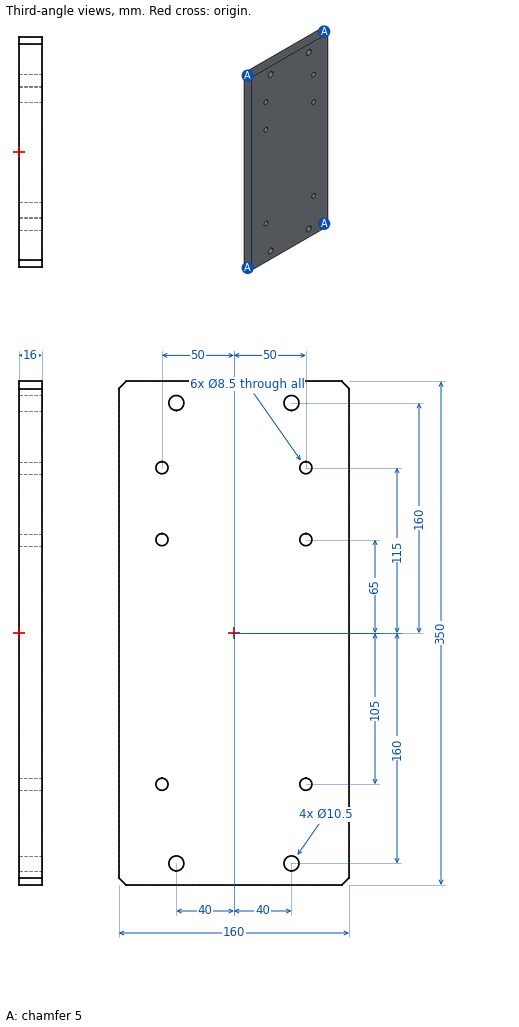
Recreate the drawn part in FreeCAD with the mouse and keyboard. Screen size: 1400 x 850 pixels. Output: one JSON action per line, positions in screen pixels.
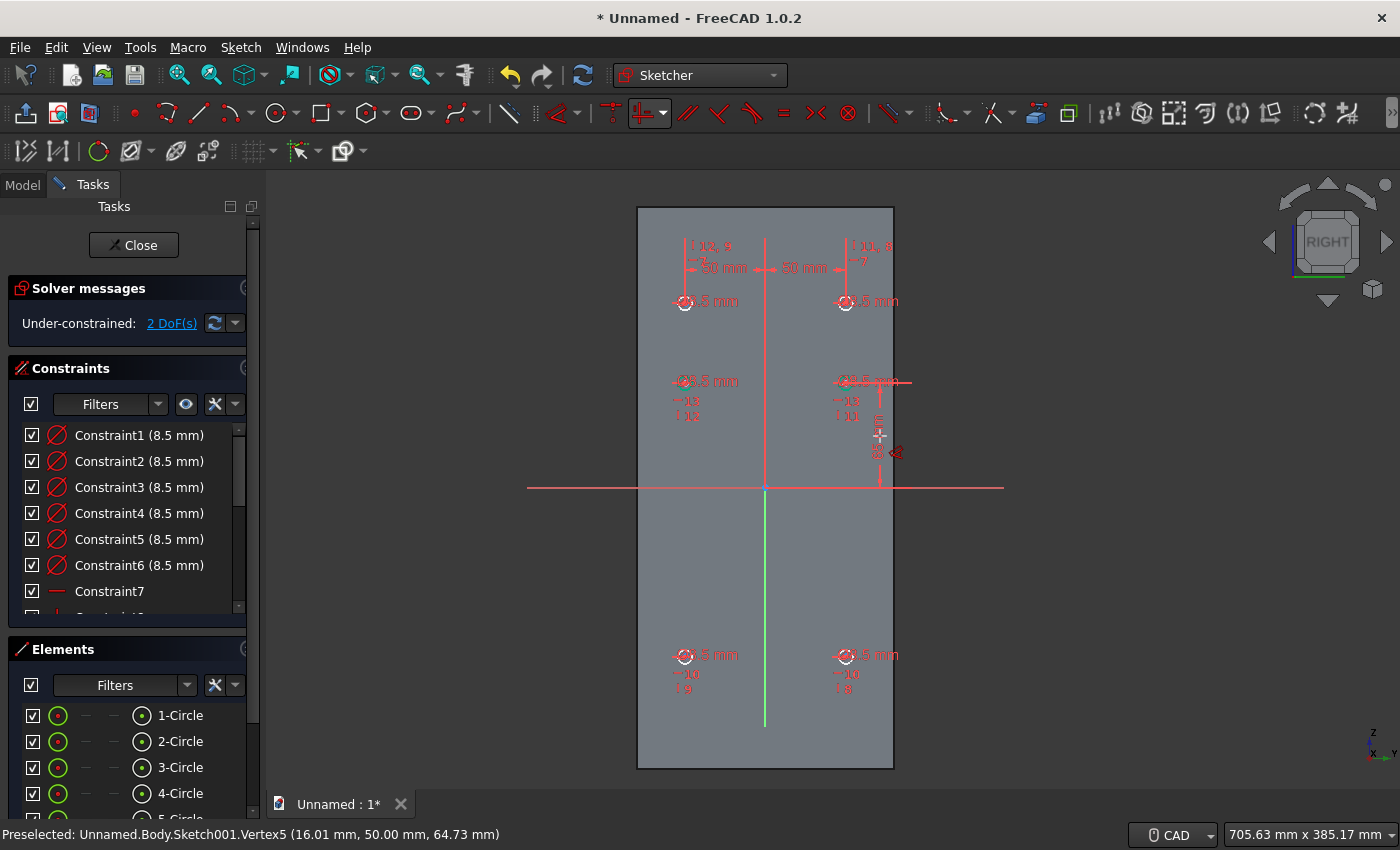
{"action": "left_click", "coordinate": [846, 303]}
{"action": "left_click", "coordinate": [880, 396]}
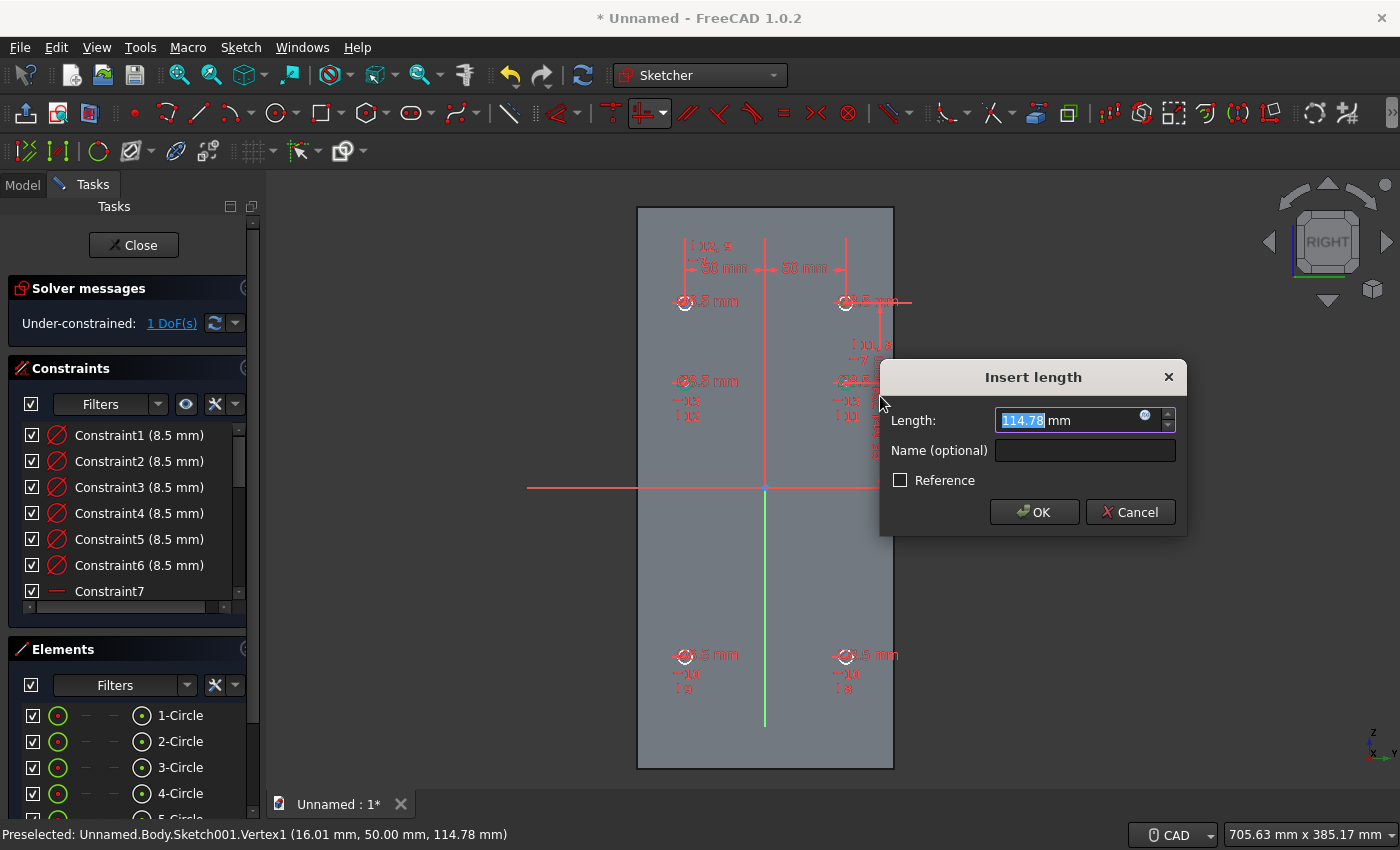
{"action": "type", "text": "115"}
{"action": "key", "text": "Return"}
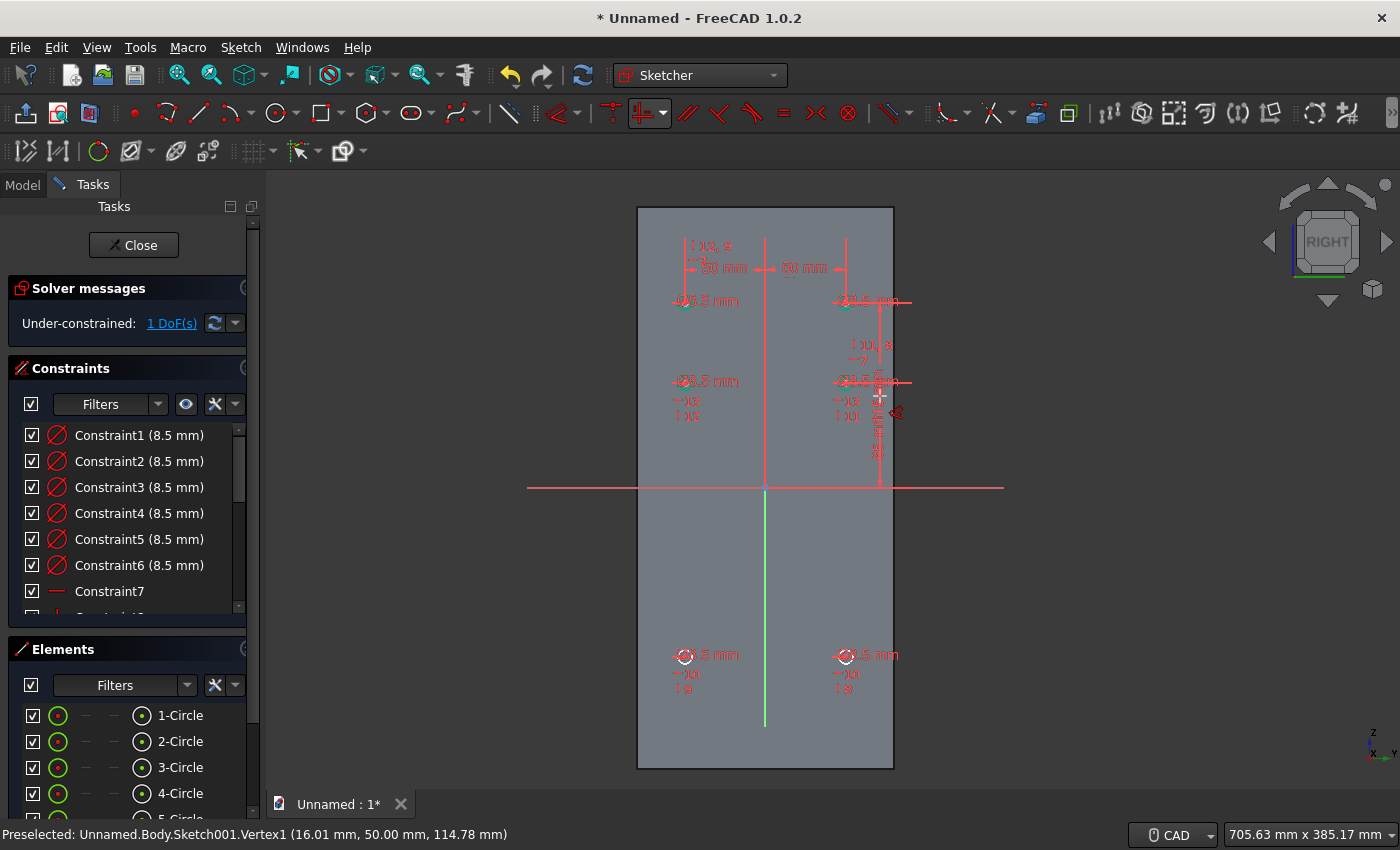
{"action": "left_click", "coordinate": [846, 657]}
{"action": "left_click", "coordinate": [880, 572]}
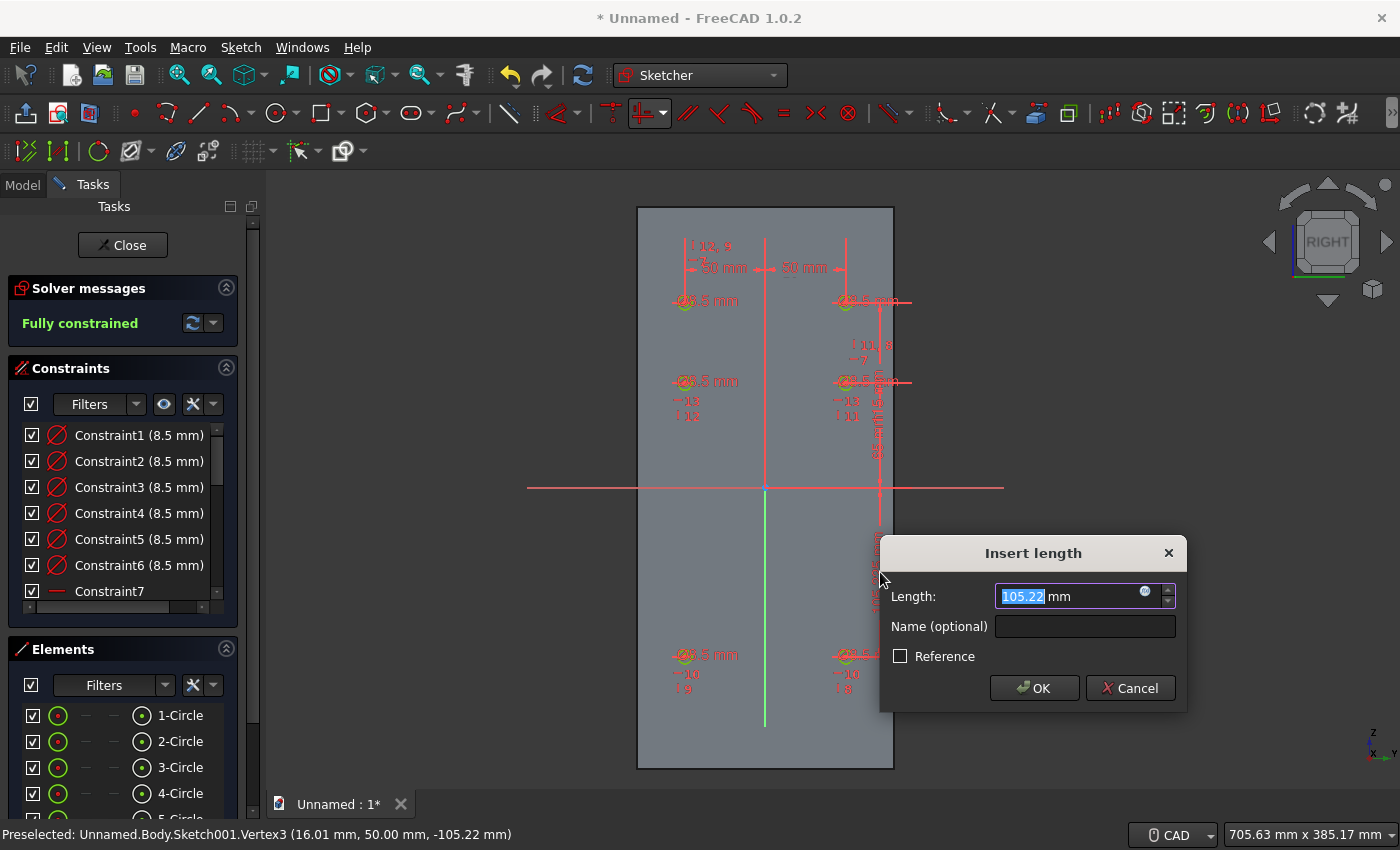
{"action": "type", "text": "105"}
{"action": "key", "text": "Return"}
{"action": "key", "text": "Escape"}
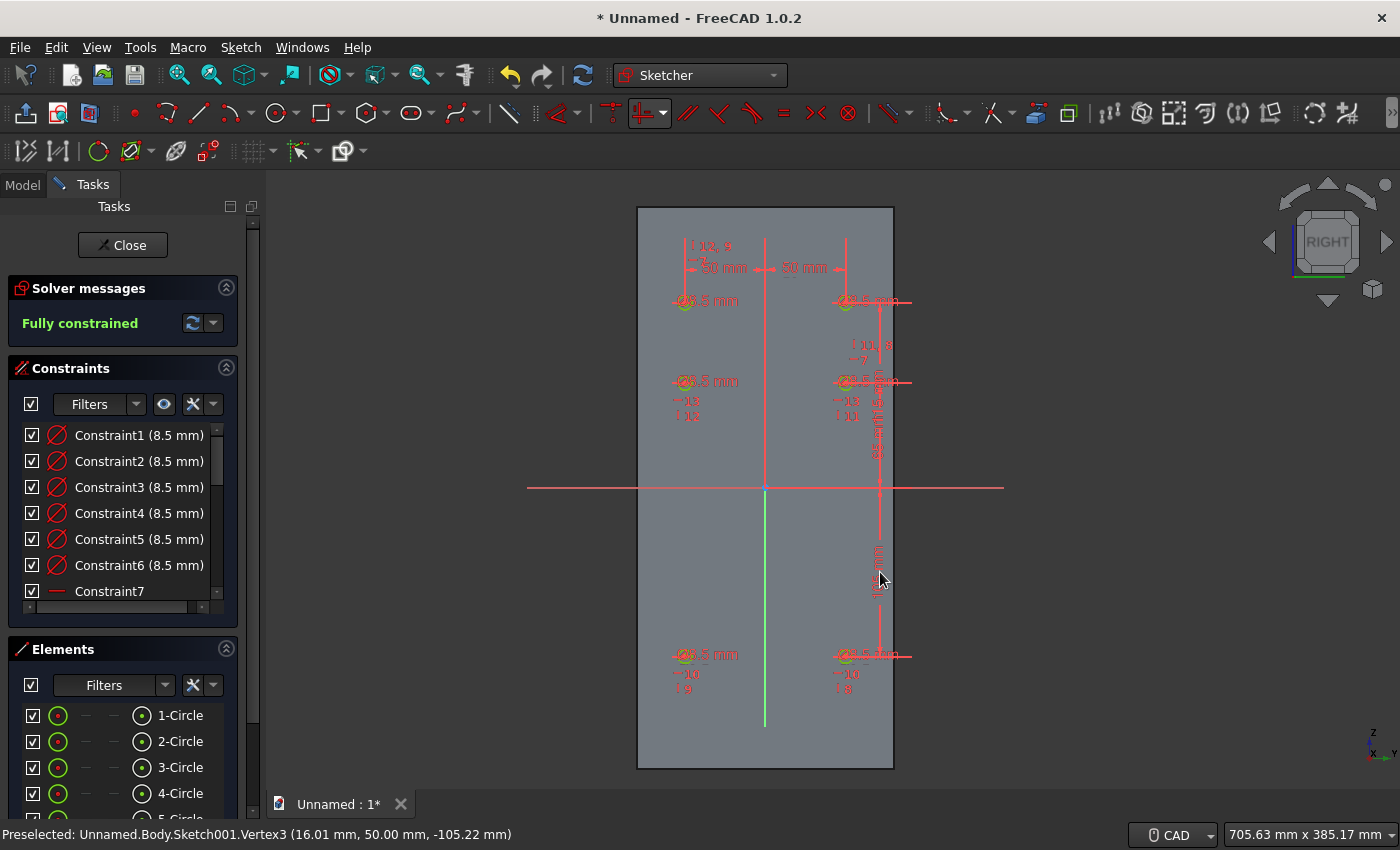
{"action": "left_click", "coordinate": [123, 245]}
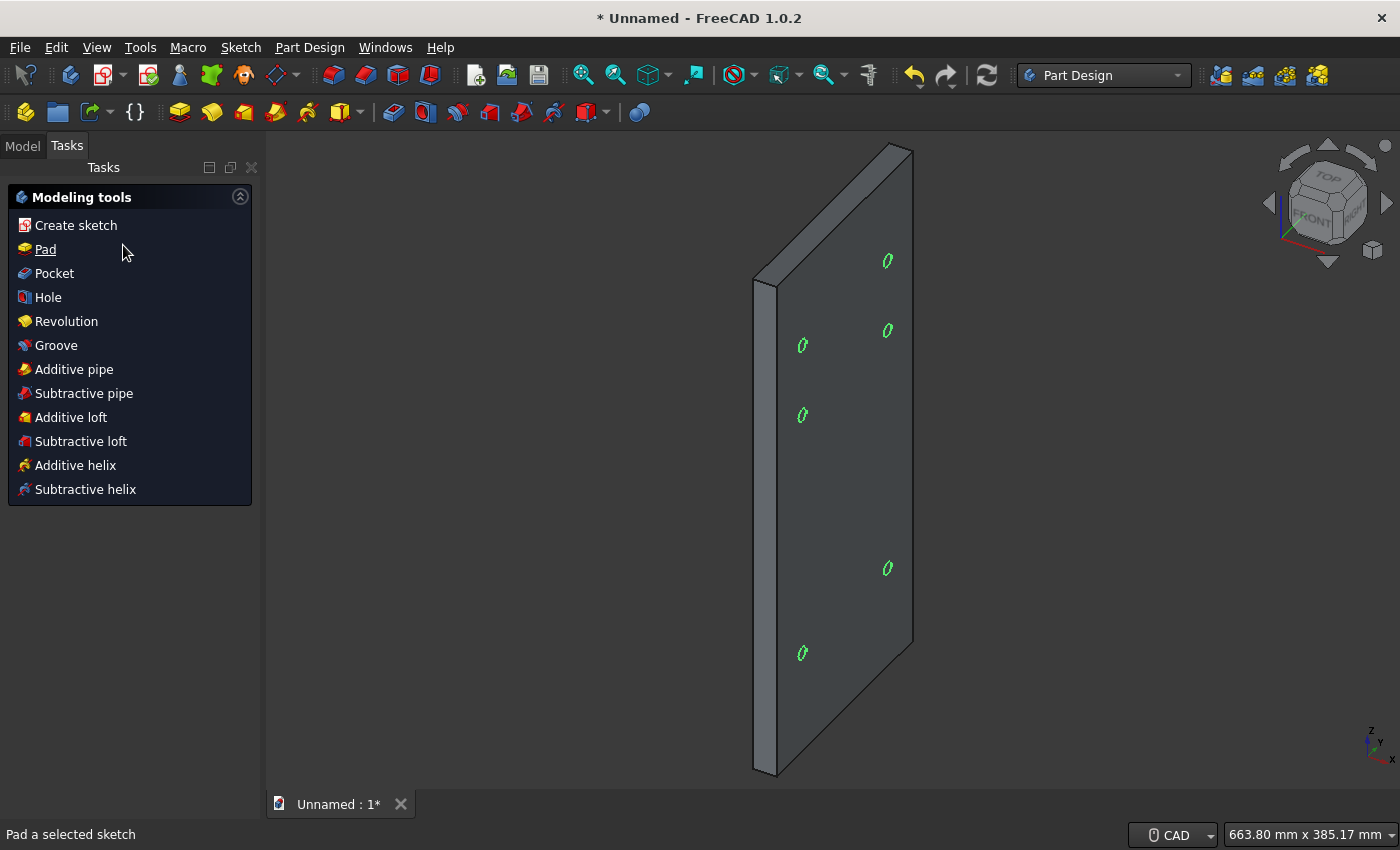
{"action": "left_click", "coordinate": [426, 112]}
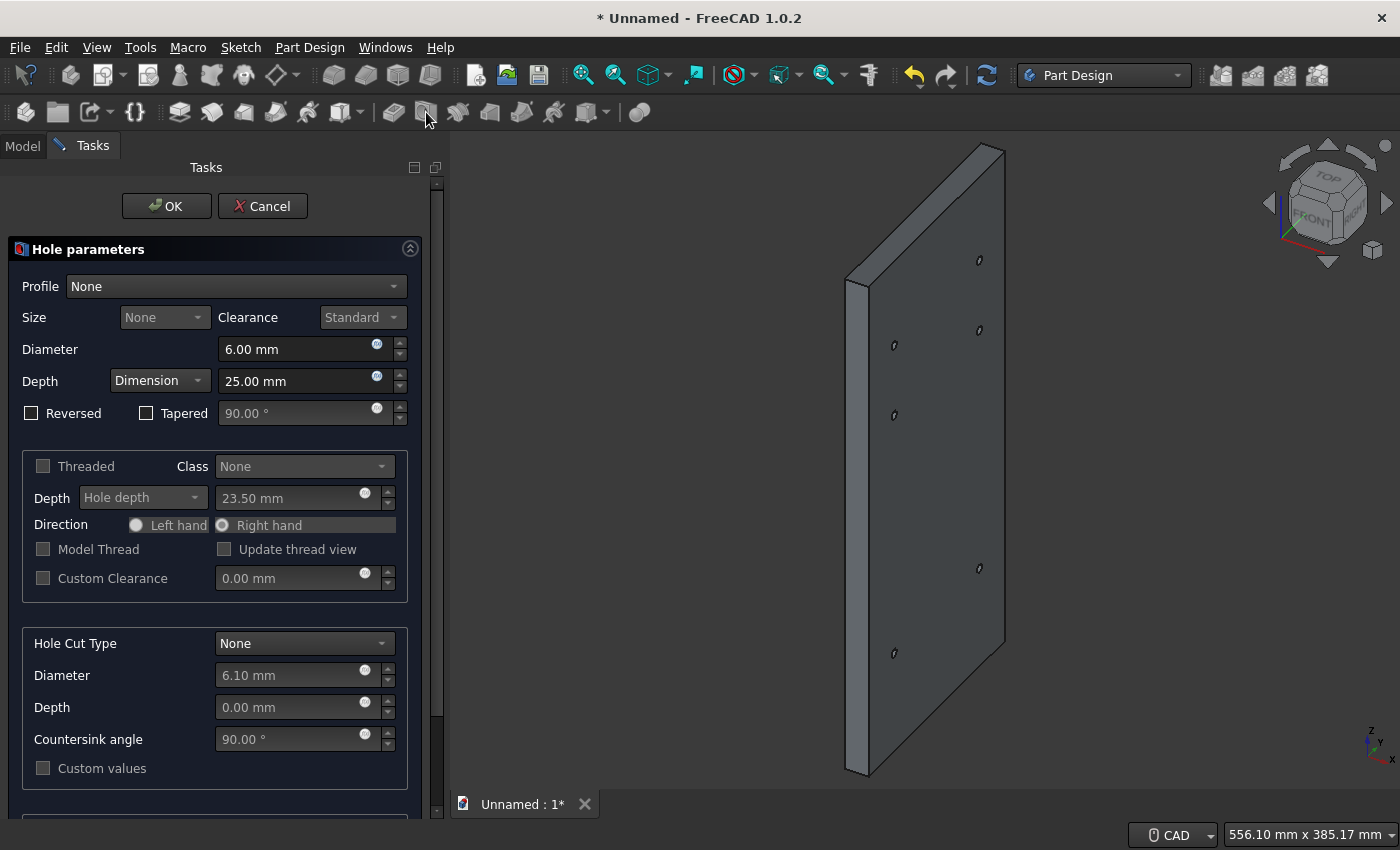
{"action": "triple_click", "coordinate": [305, 349]}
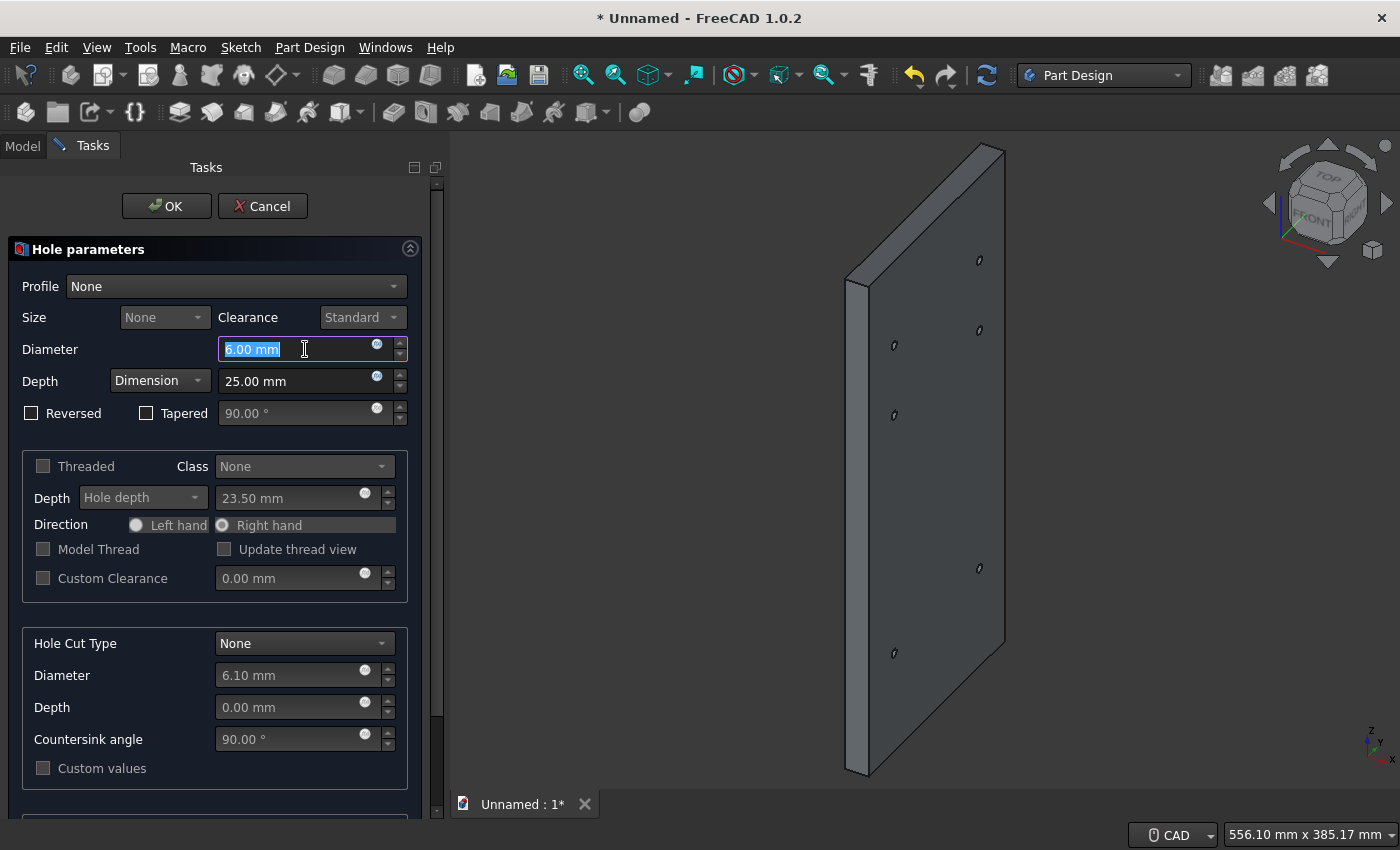
{"action": "type", "text": "8.5"}
{"action": "key", "text": "Tab"}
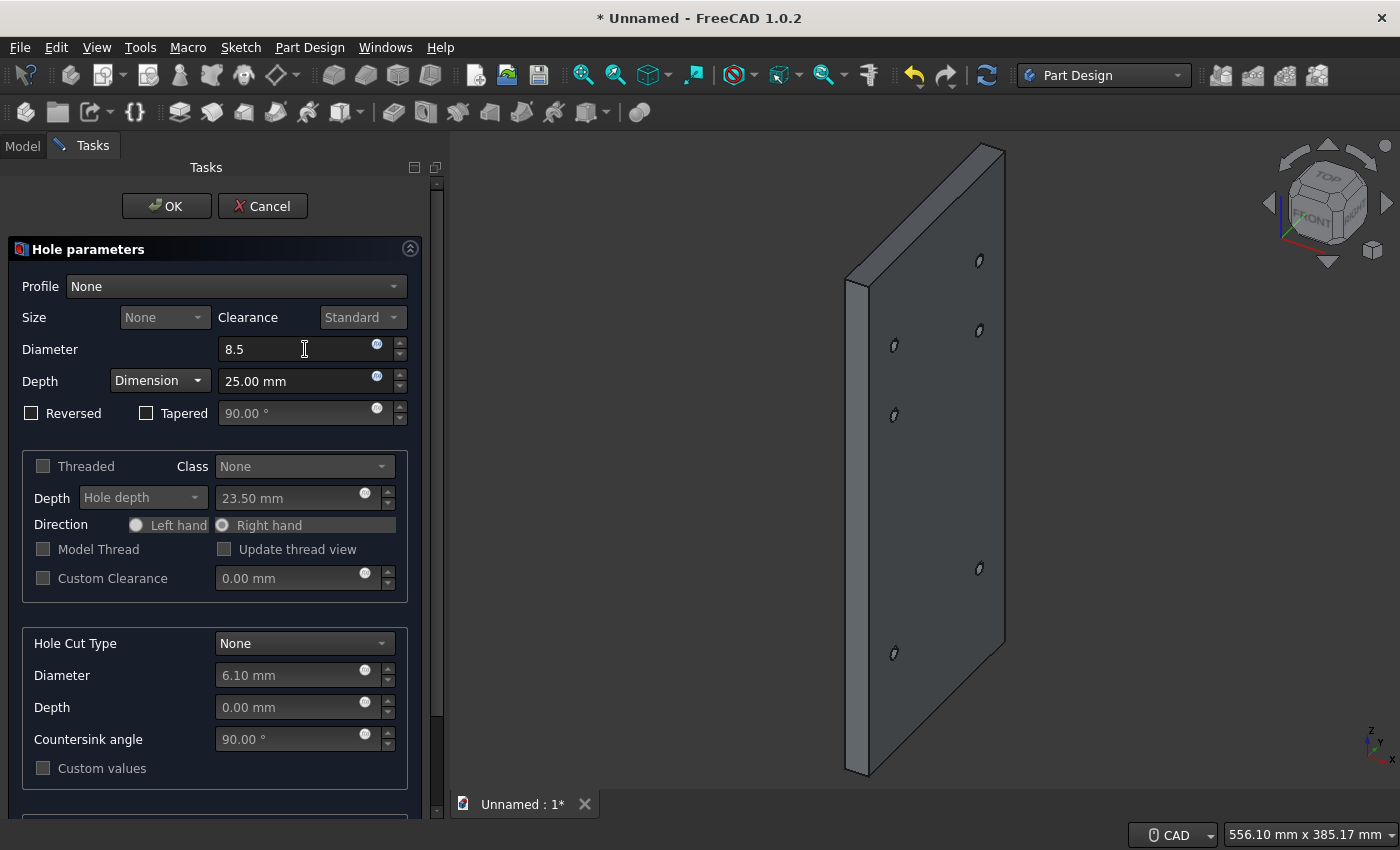
{"action": "left_click", "coordinate": [161, 380]}